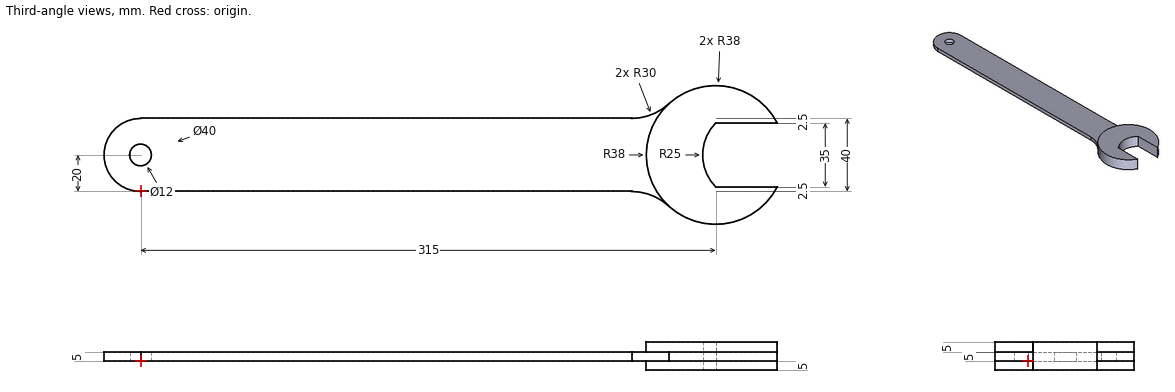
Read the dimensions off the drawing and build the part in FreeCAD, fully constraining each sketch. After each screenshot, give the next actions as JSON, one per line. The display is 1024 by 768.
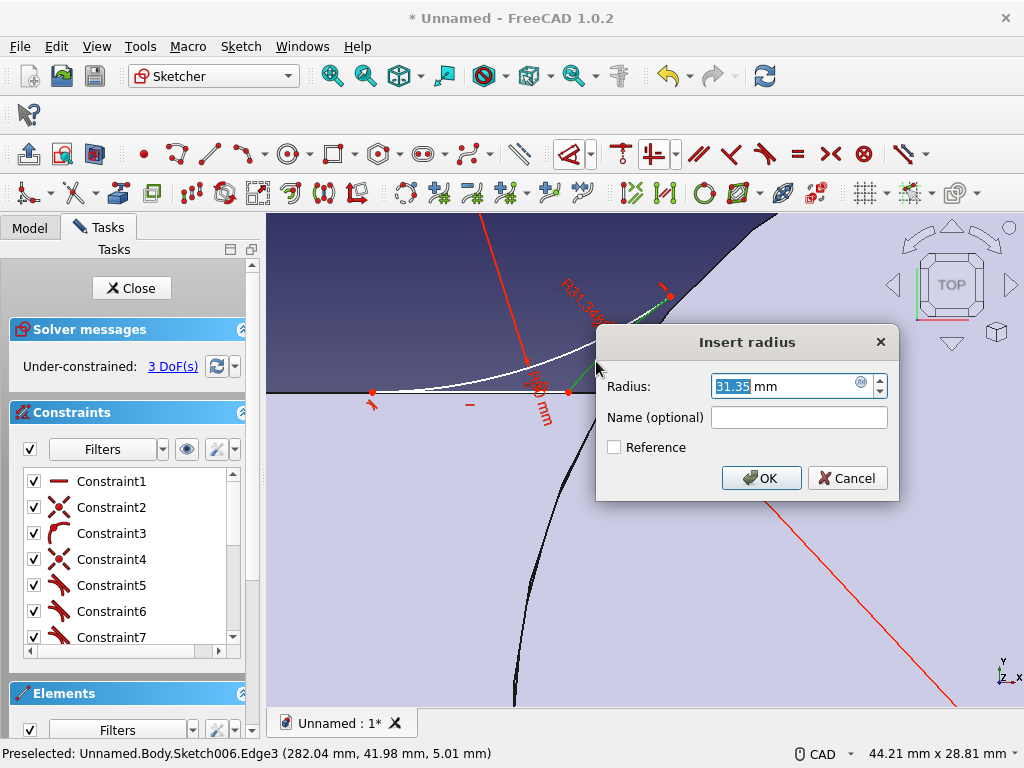
{"action": "type", "text": "38"}
{"action": "key", "text": "Return"}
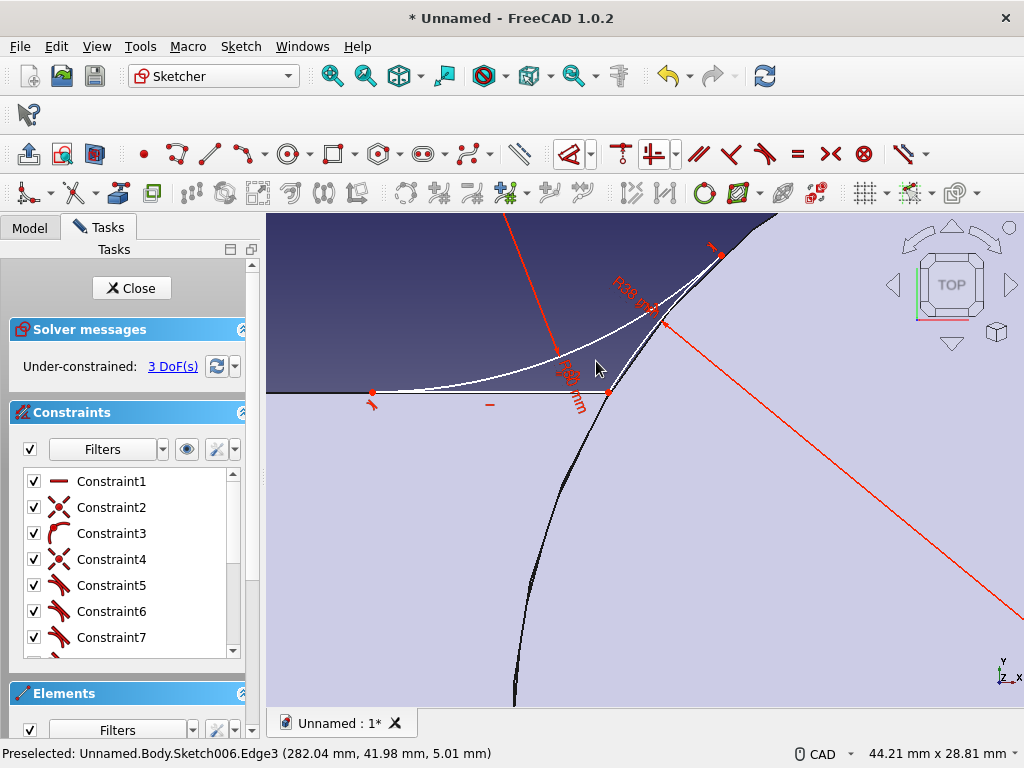
{"action": "left_click", "coordinate": [609, 392]}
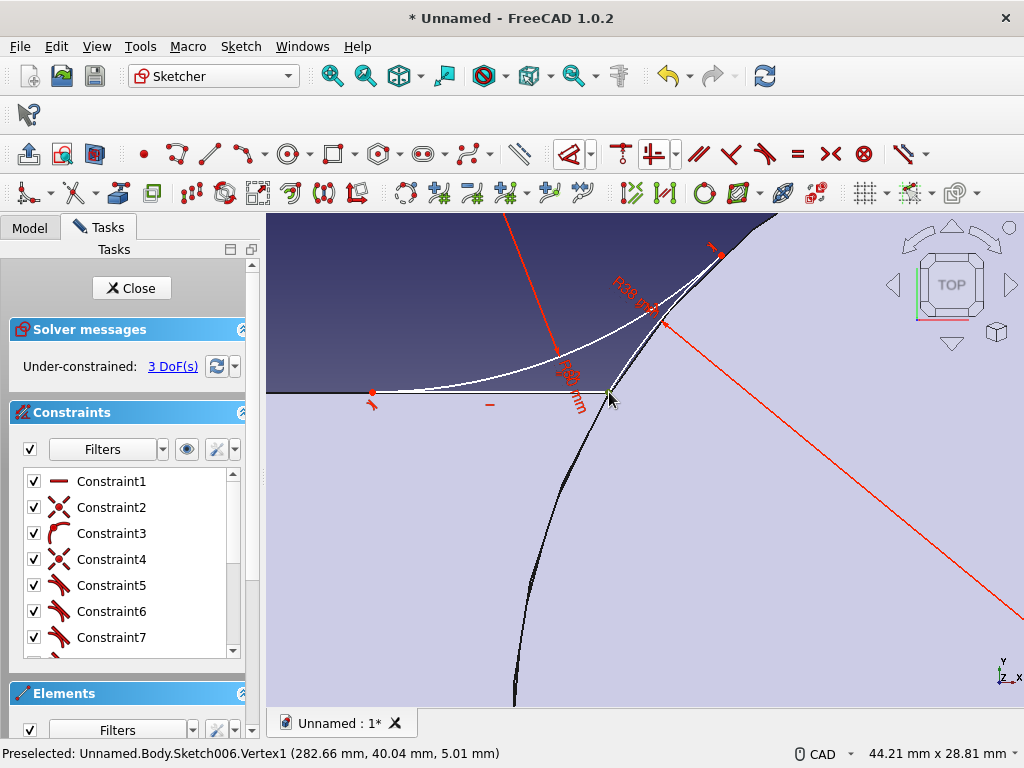
{"action": "key", "text": "i"}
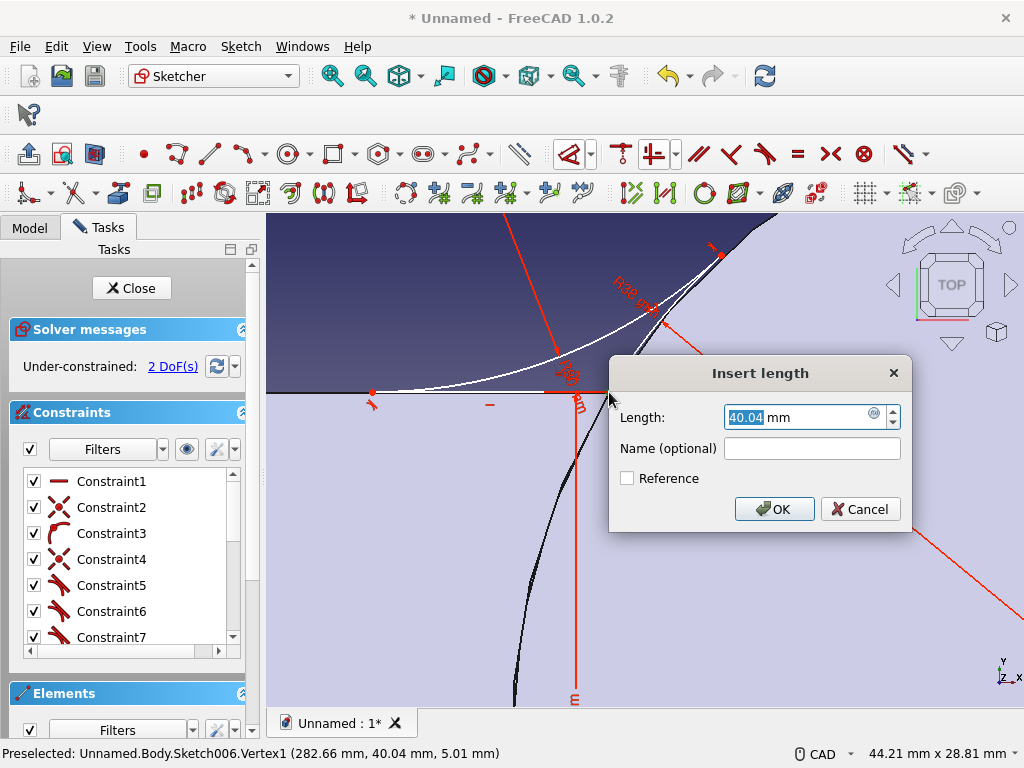
{"action": "type", "text": "40"}
{"action": "key", "text": "Return"}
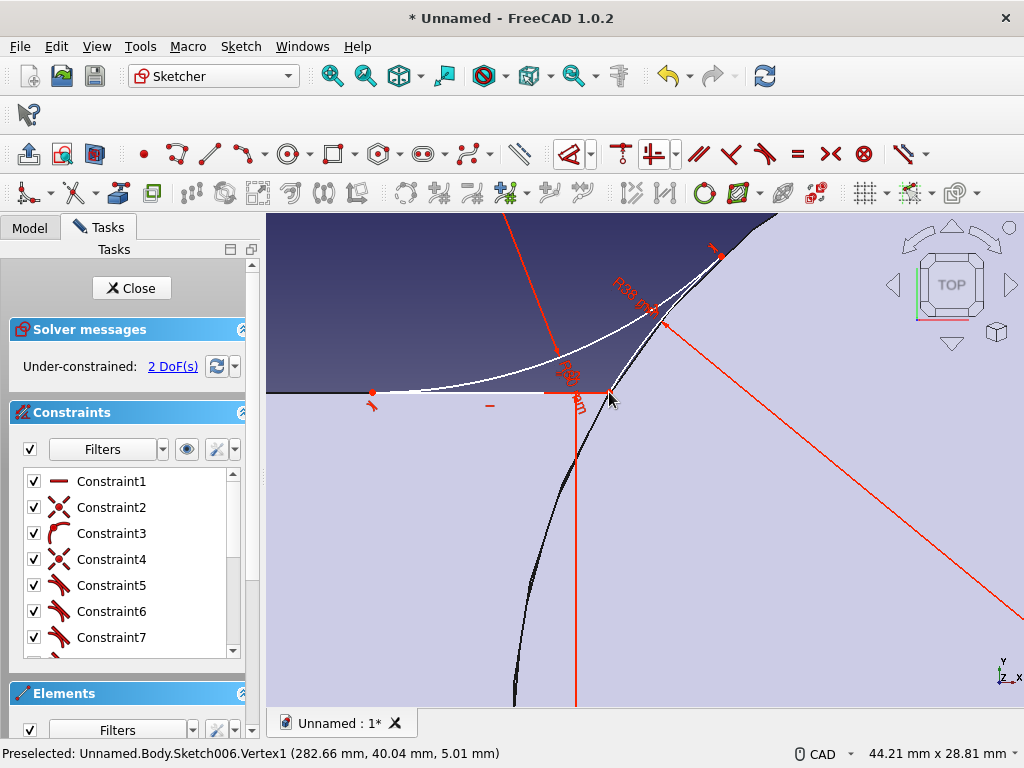
{"action": "scroll", "coordinate": [589, 341], "scroll_direction": "down", "scroll_amount": 6}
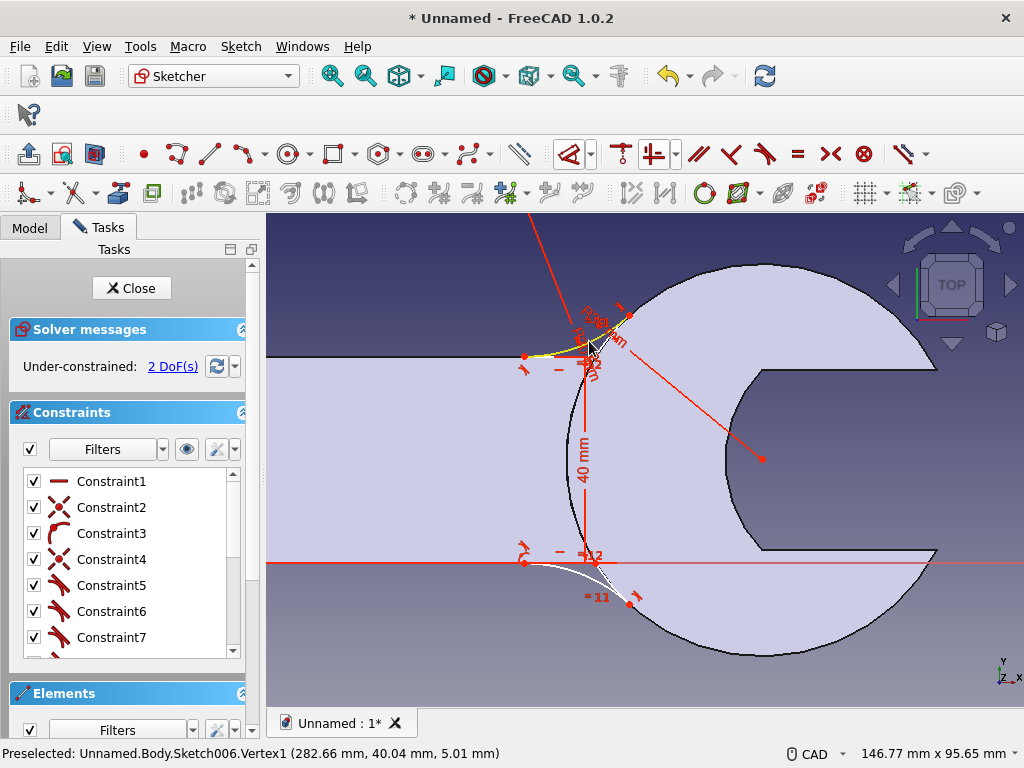
{"action": "left_click", "coordinate": [762, 460]}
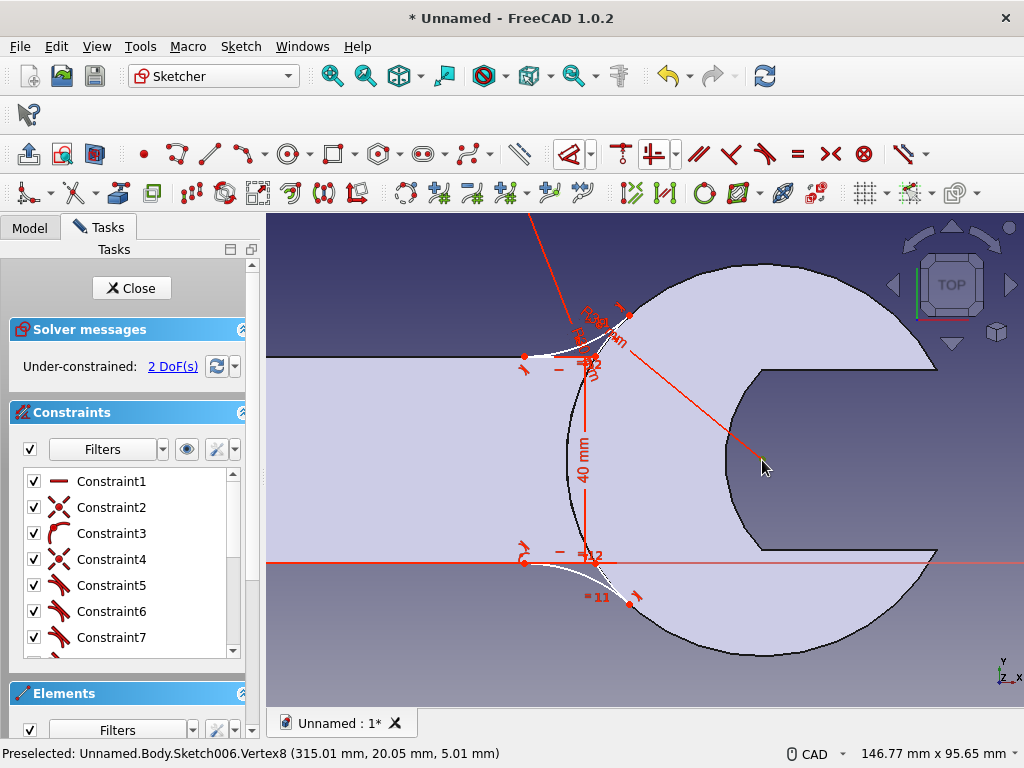
{"action": "key", "text": "i"}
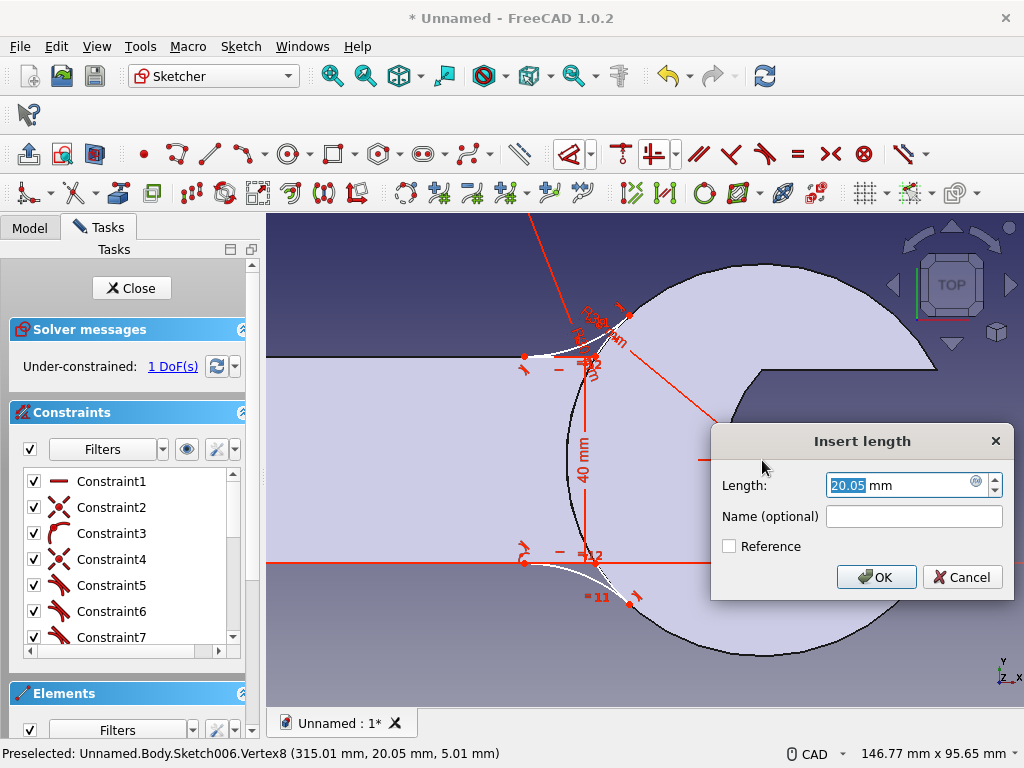
{"action": "type", "text": "20"}
{"action": "key", "text": "Return"}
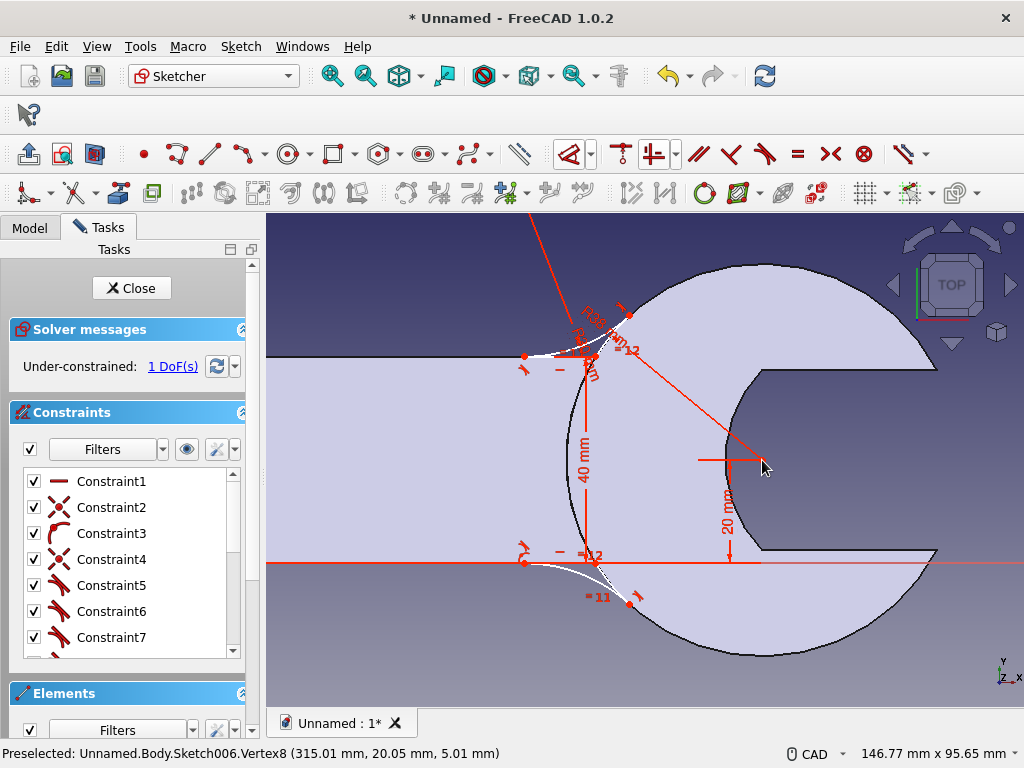
{"action": "left_click", "coordinate": [763, 460]}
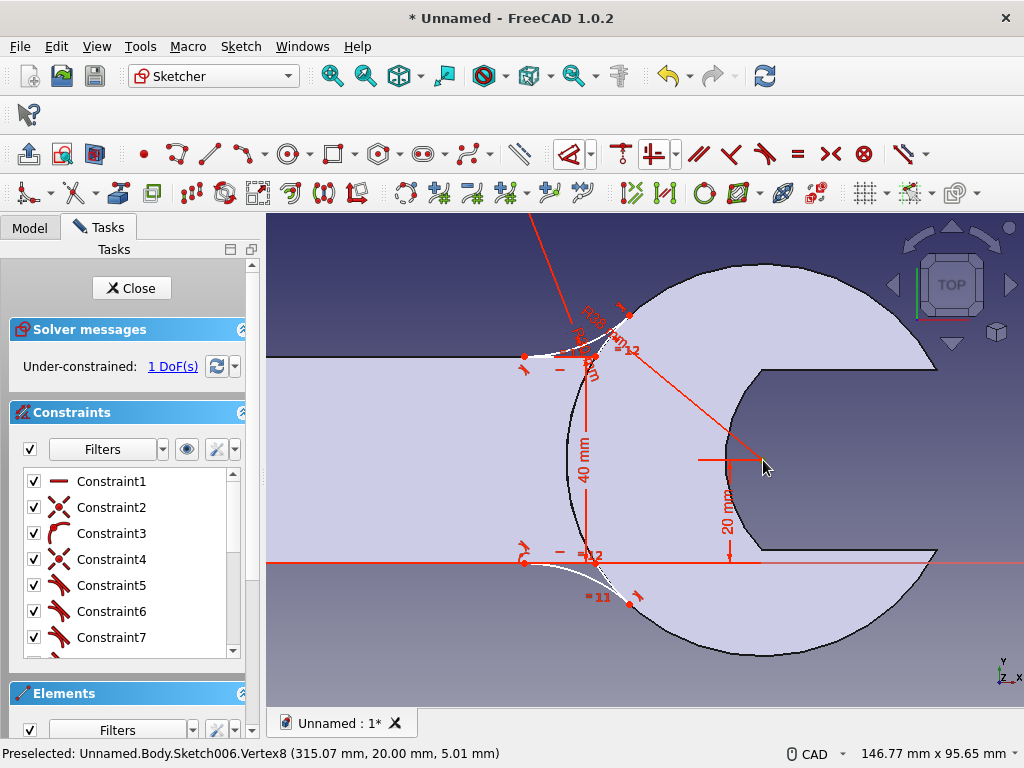
{"action": "key", "text": "l"}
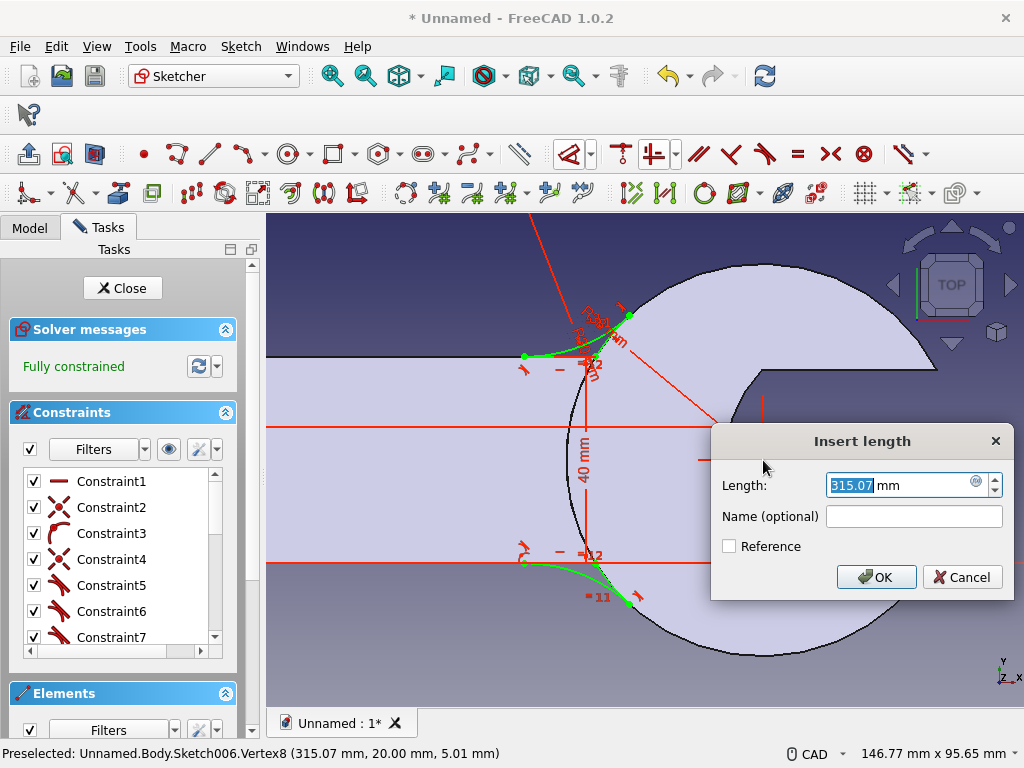
{"action": "type", "text": "315"}
{"action": "key", "text": "Return"}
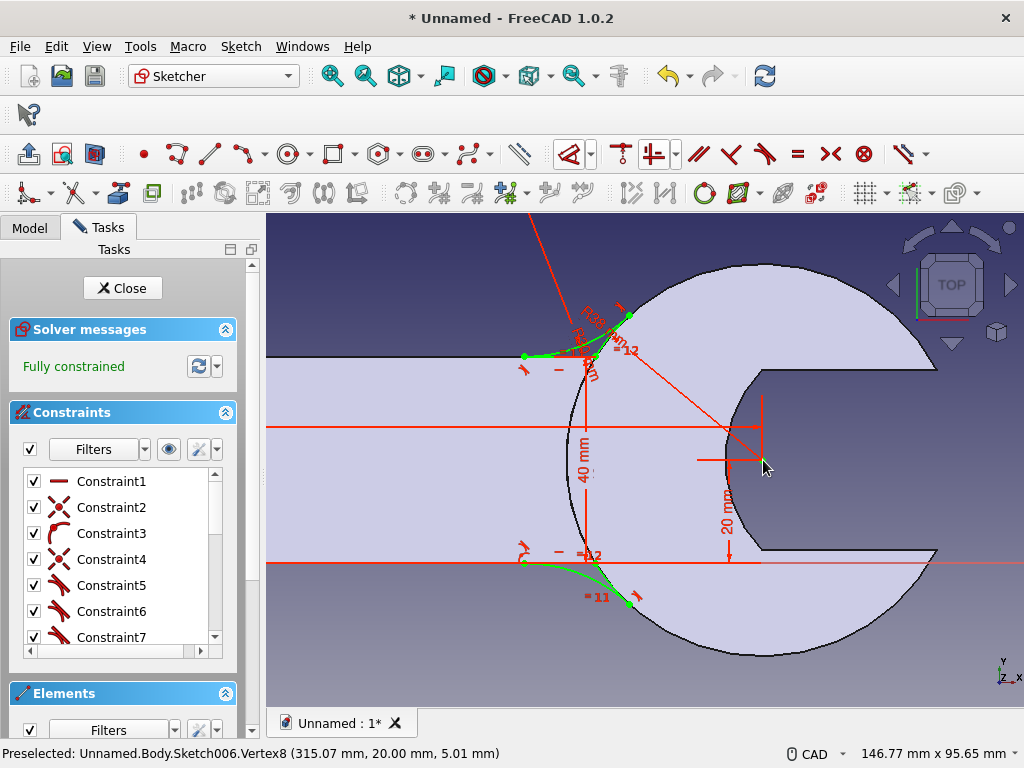
{"action": "left_click", "coordinate": [123, 288]}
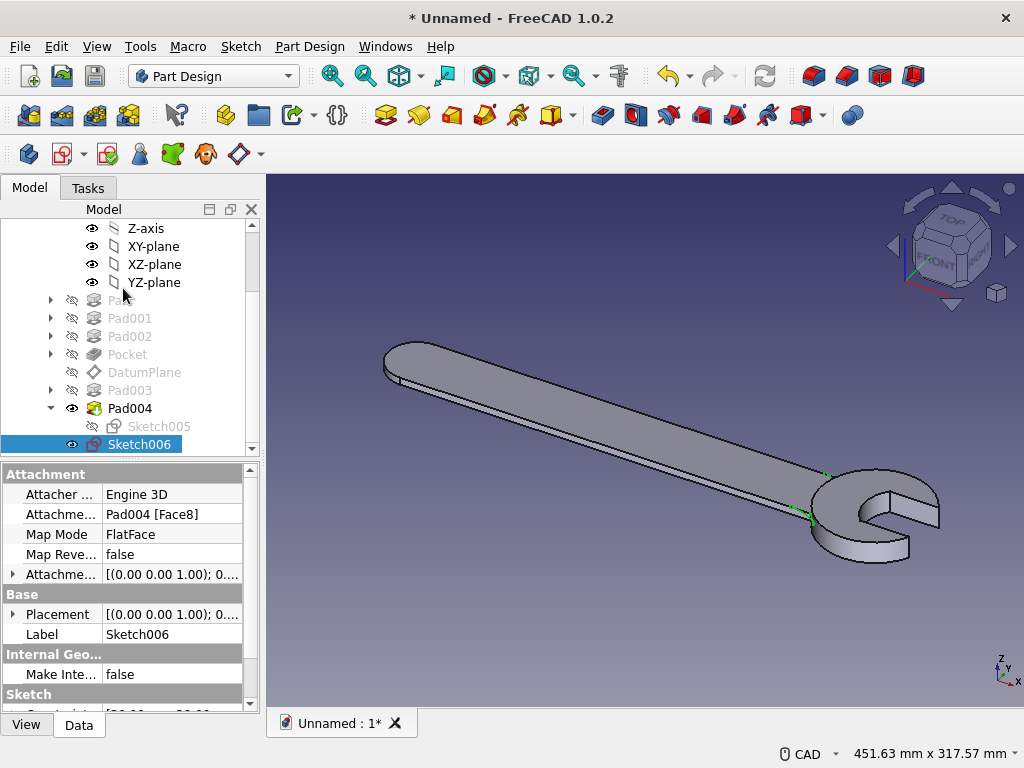
{"action": "left_click", "coordinate": [386, 116]}